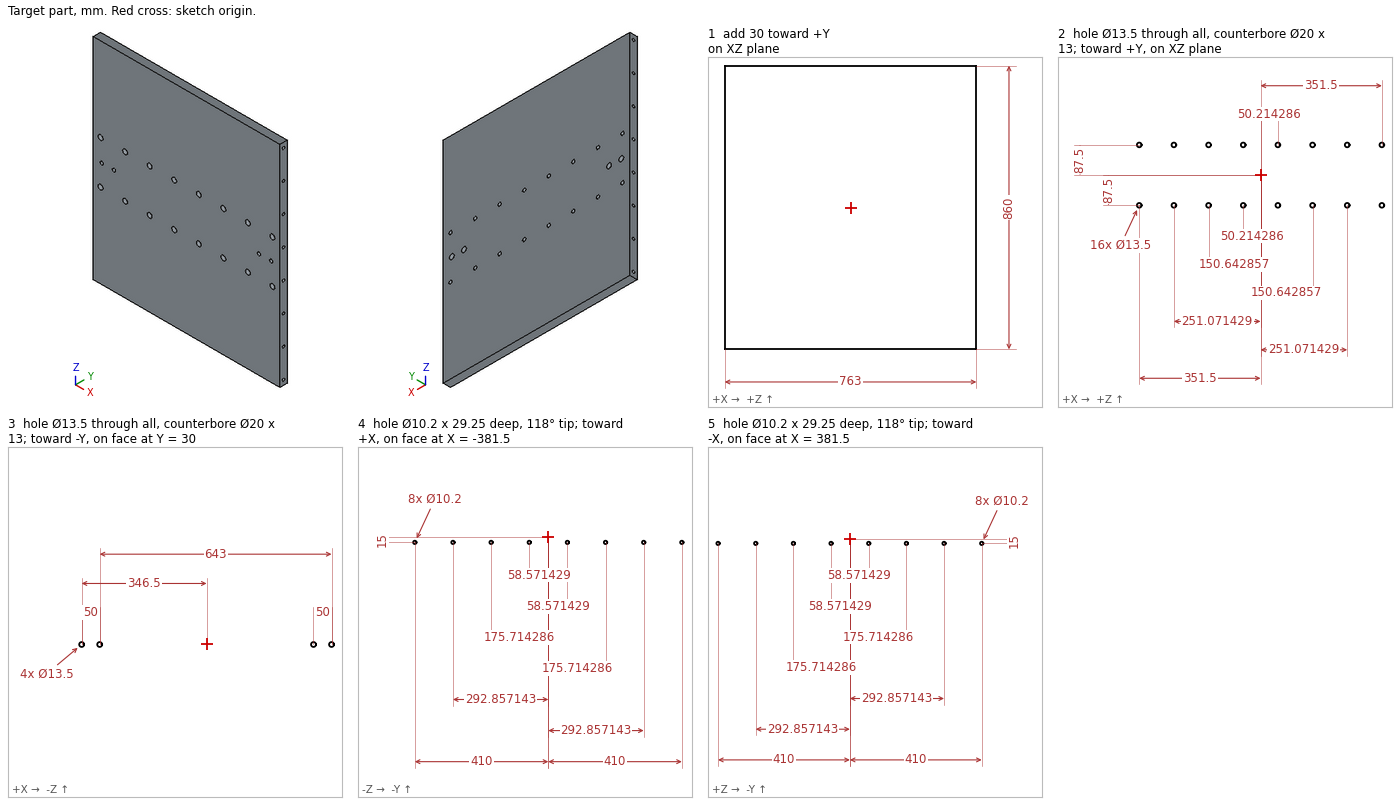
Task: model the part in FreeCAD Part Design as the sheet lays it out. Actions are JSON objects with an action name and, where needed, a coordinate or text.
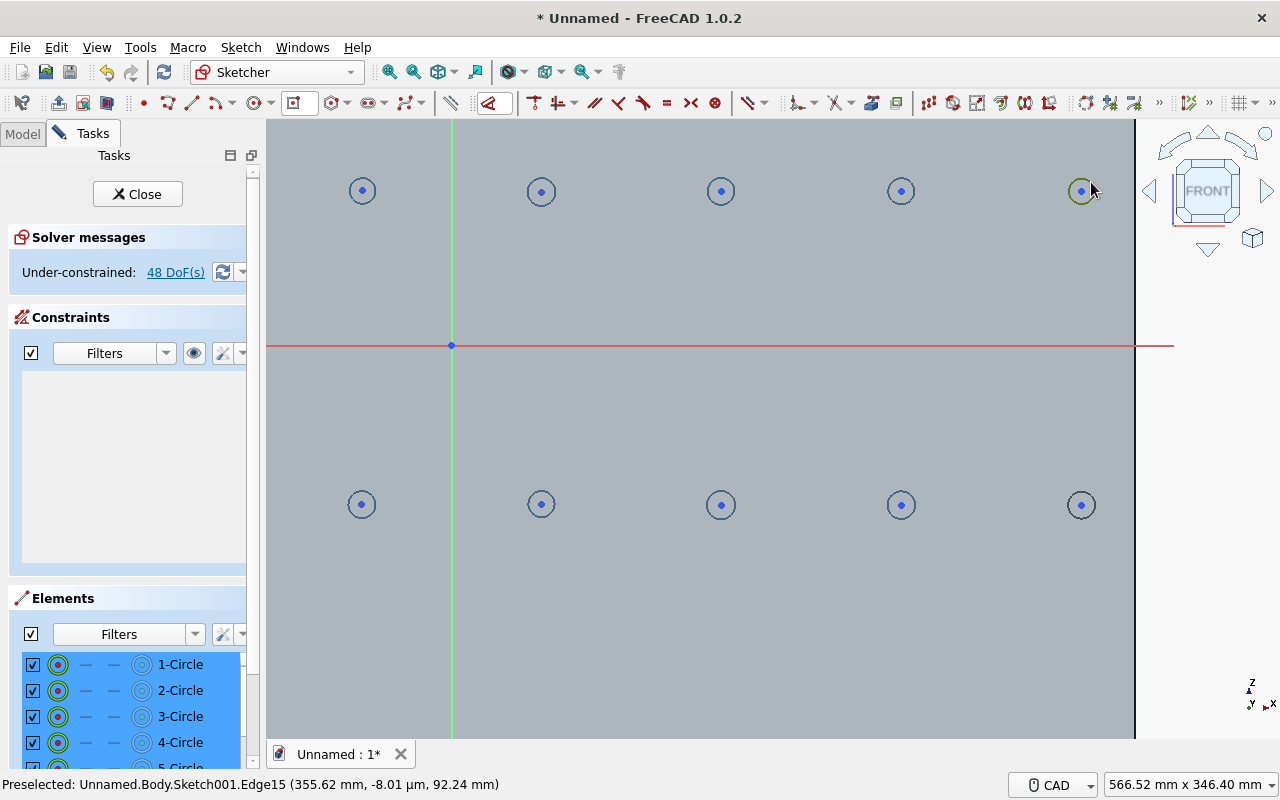
{"action": "left_click", "coordinate": [1091, 496]}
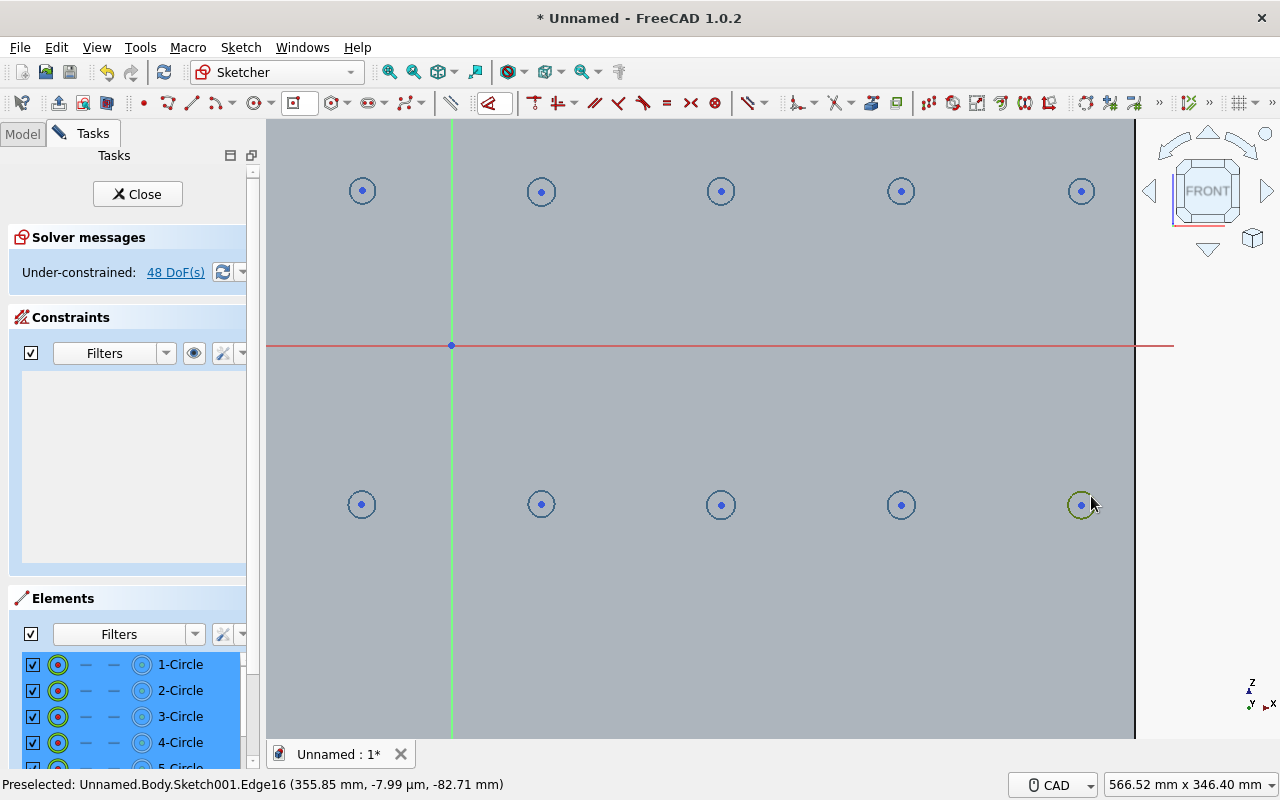
{"action": "left_click", "coordinate": [668, 104]}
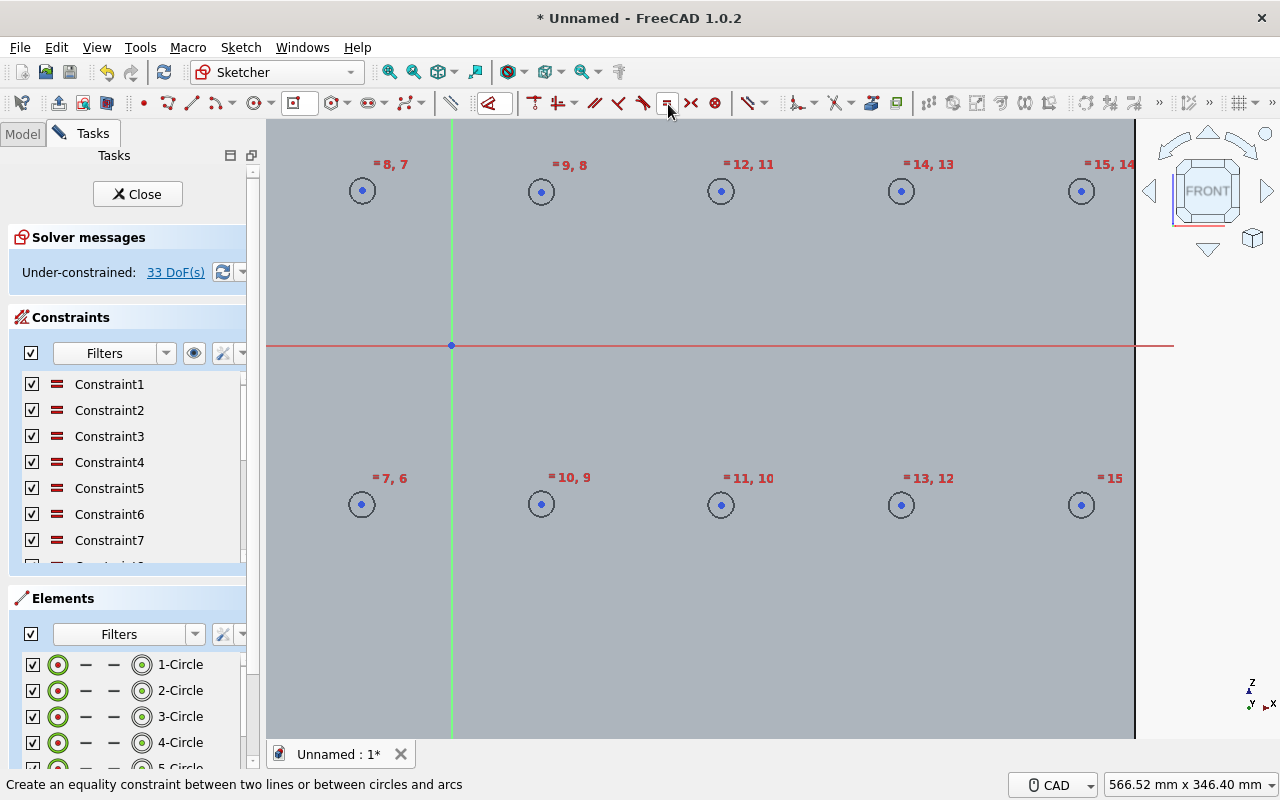
{"action": "scroll", "coordinate": [911, 497], "scroll_direction": "down", "scroll_amount": 4}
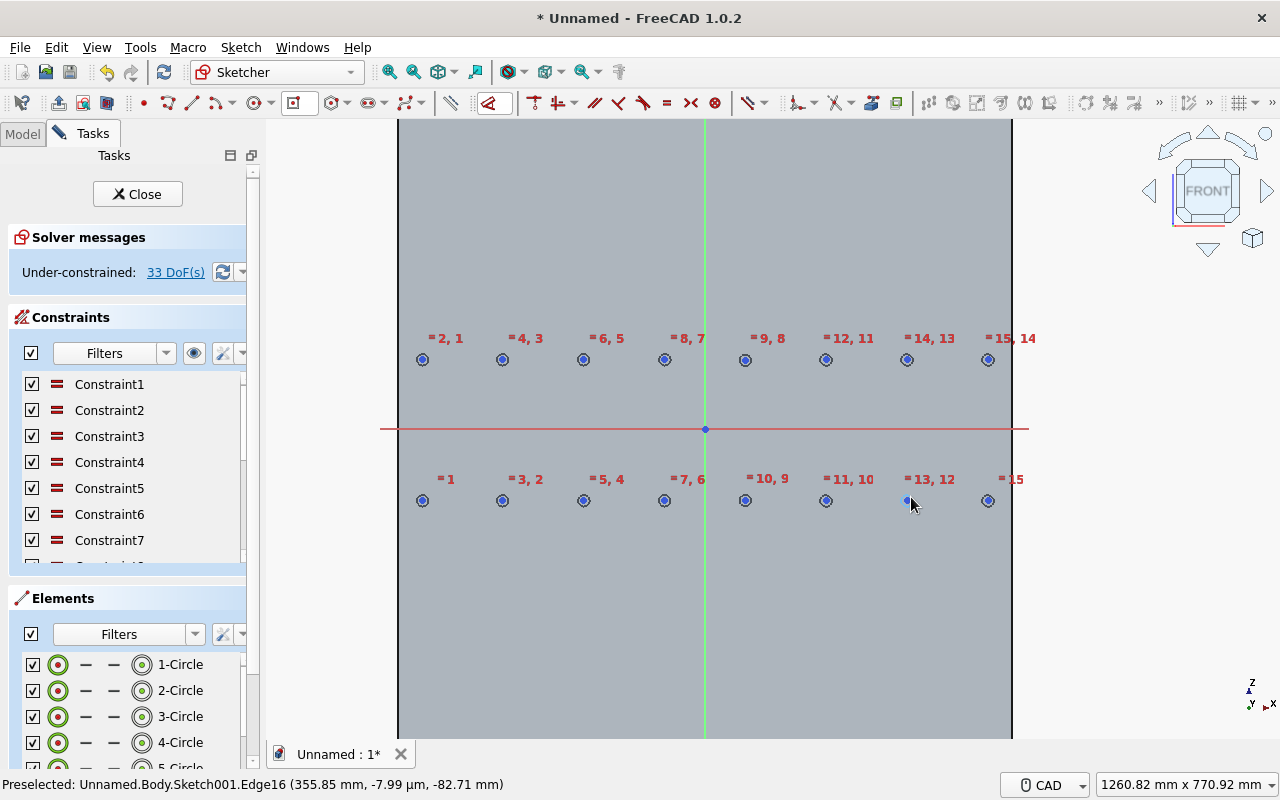
{"action": "left_click", "coordinate": [423, 501]}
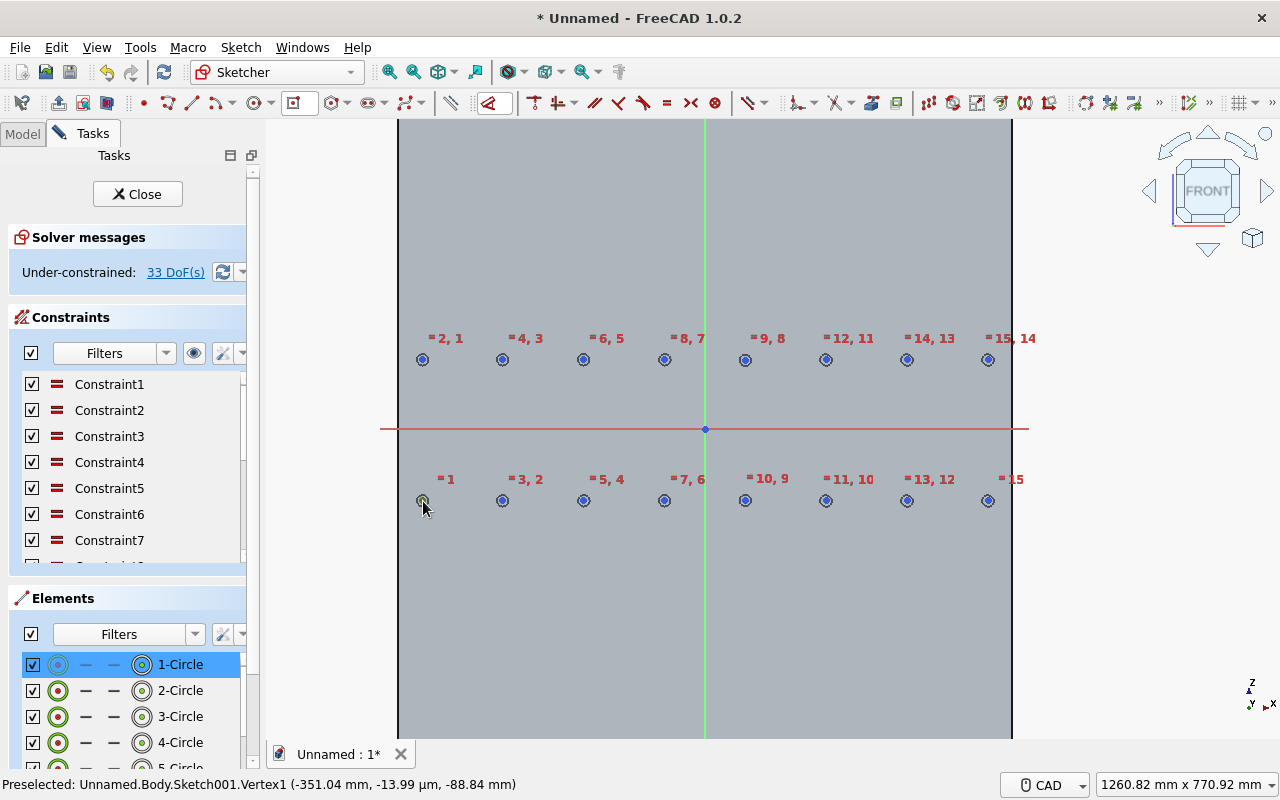
{"action": "left_click", "coordinate": [423, 360]}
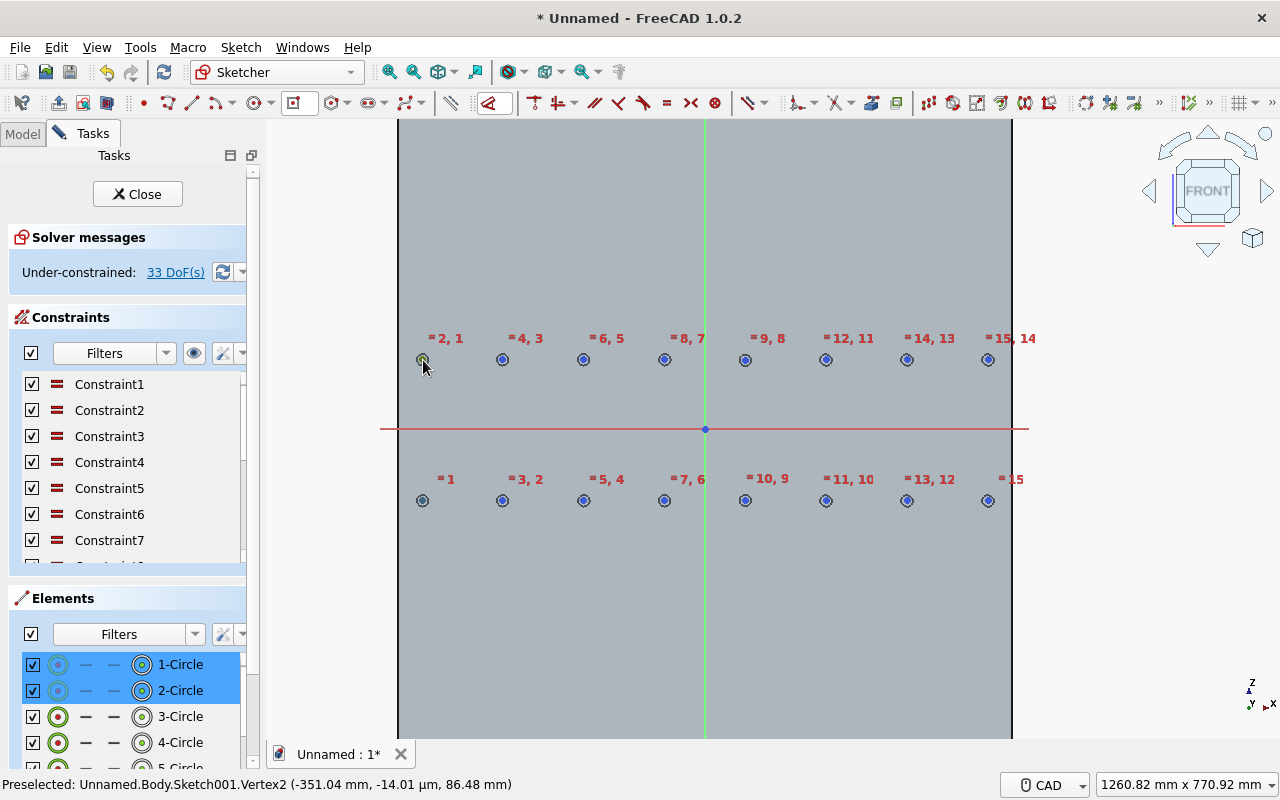
{"action": "left_click", "coordinate": [576, 104]}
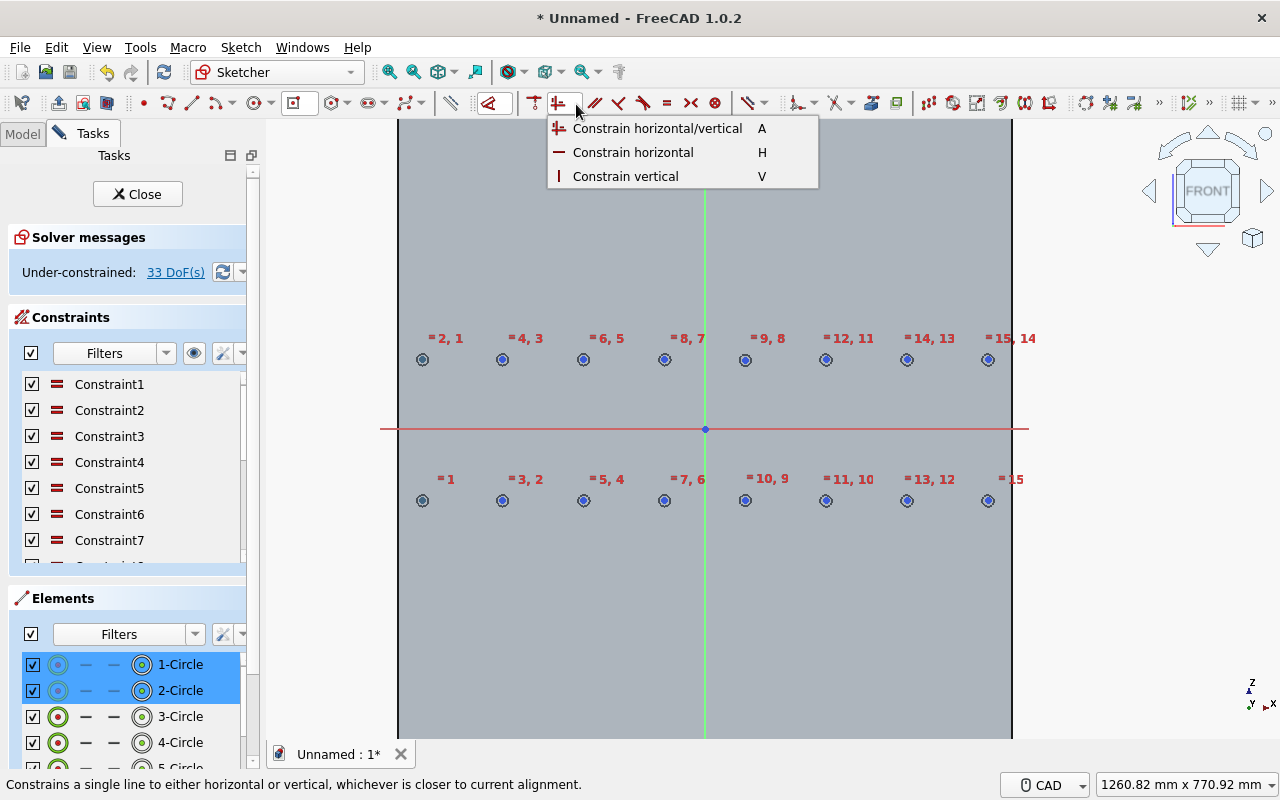
{"action": "left_click", "coordinate": [683, 176]}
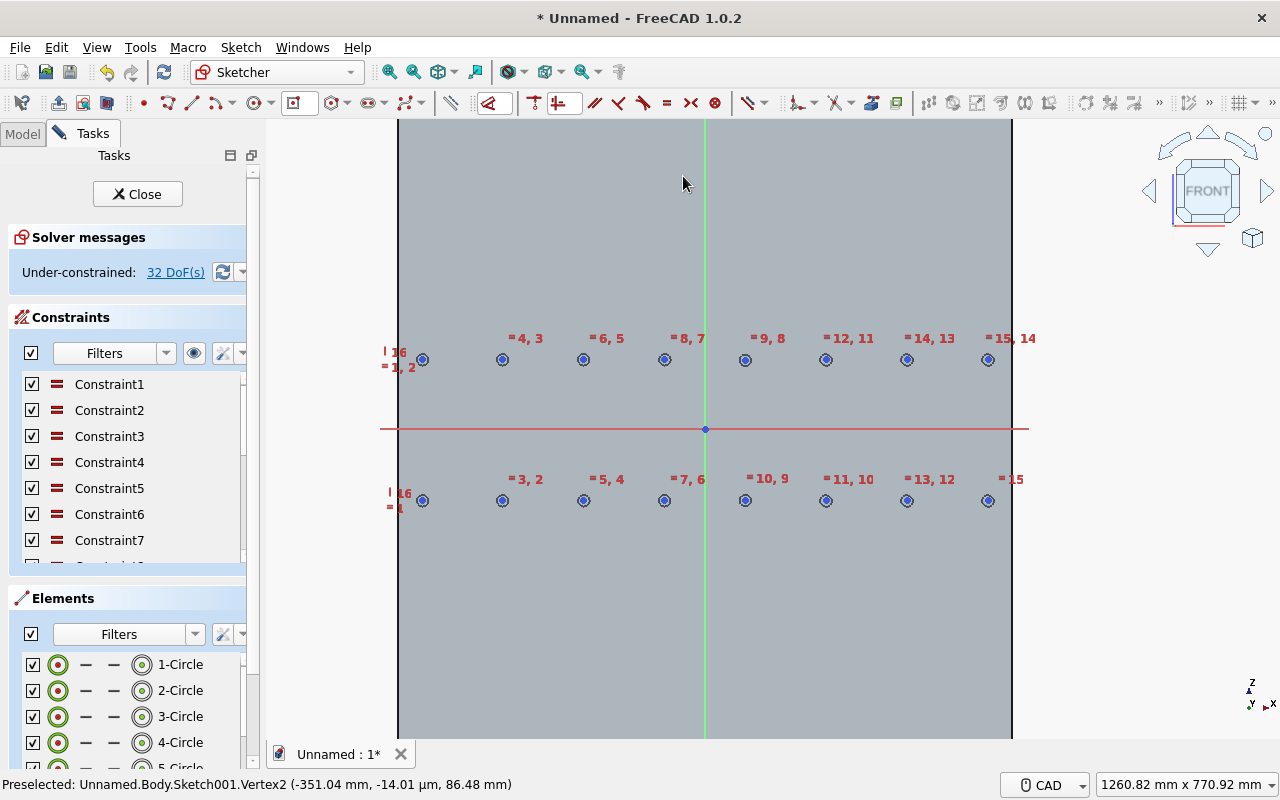
{"action": "left_click", "coordinate": [423, 501]}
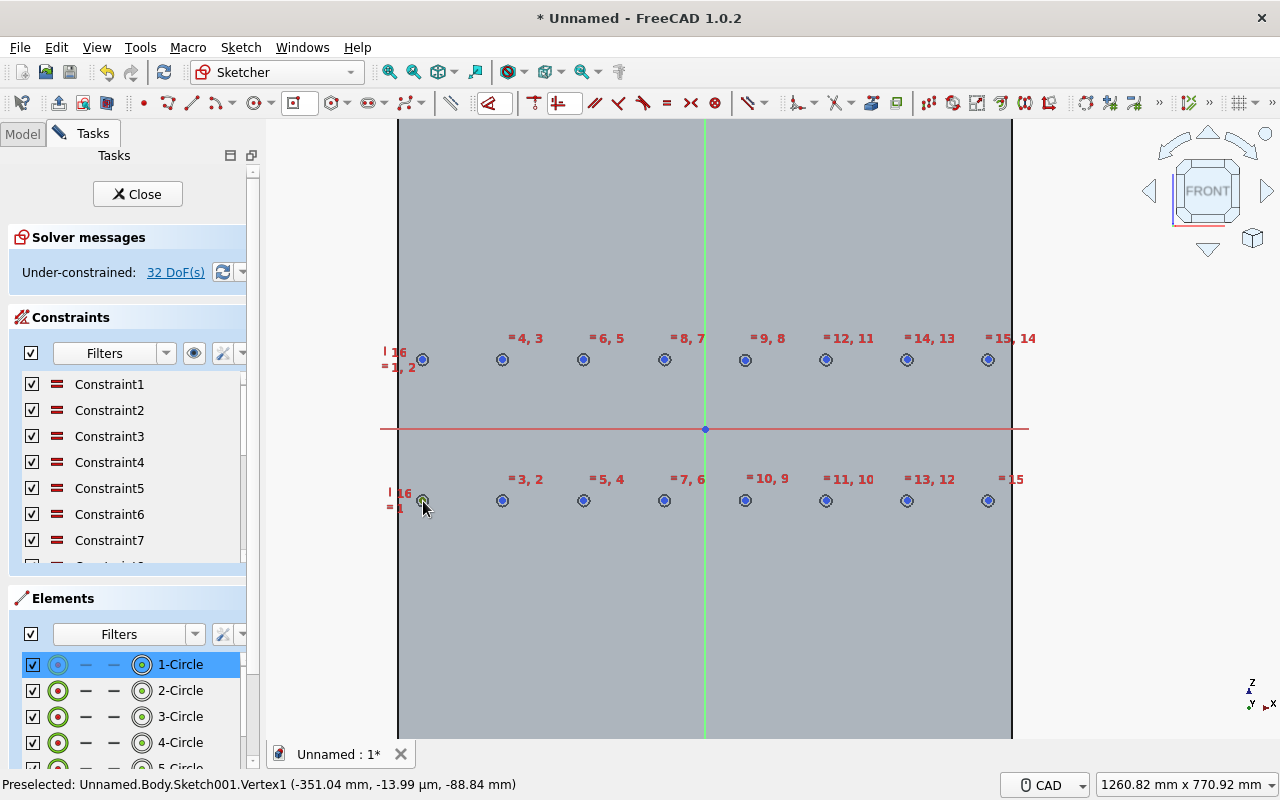
{"action": "left_click", "coordinate": [503, 501]}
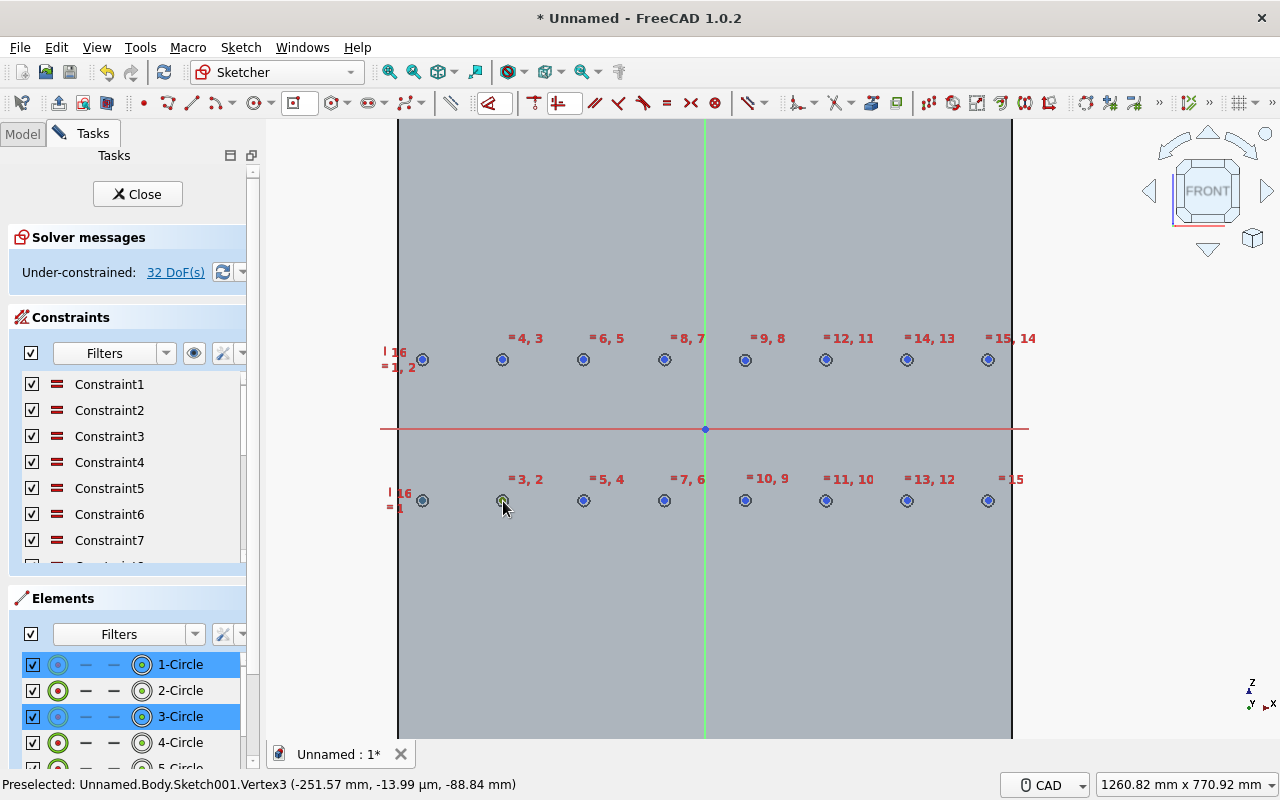
{"action": "left_click", "coordinate": [576, 104]}